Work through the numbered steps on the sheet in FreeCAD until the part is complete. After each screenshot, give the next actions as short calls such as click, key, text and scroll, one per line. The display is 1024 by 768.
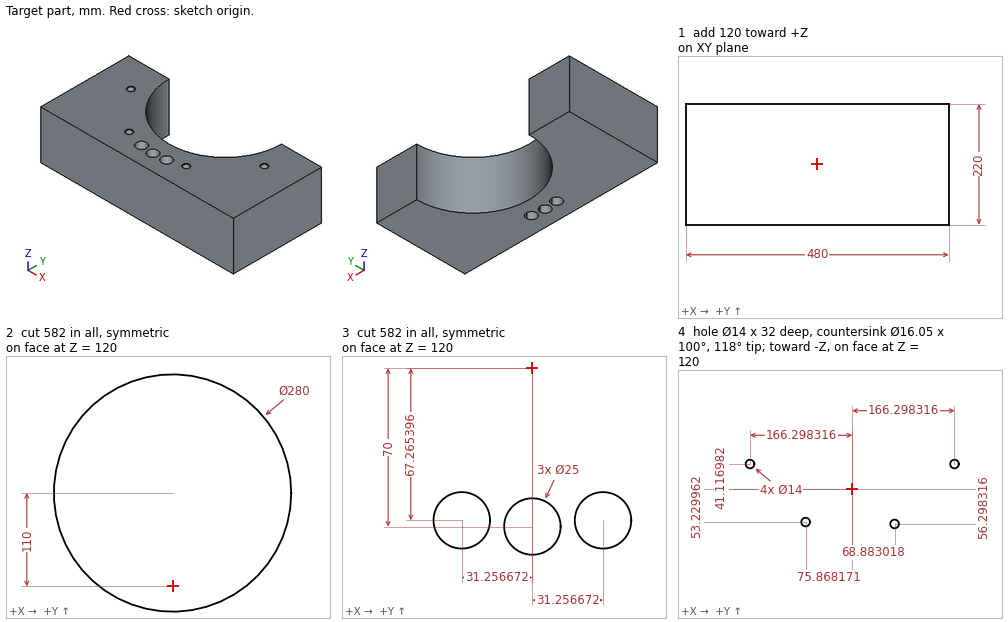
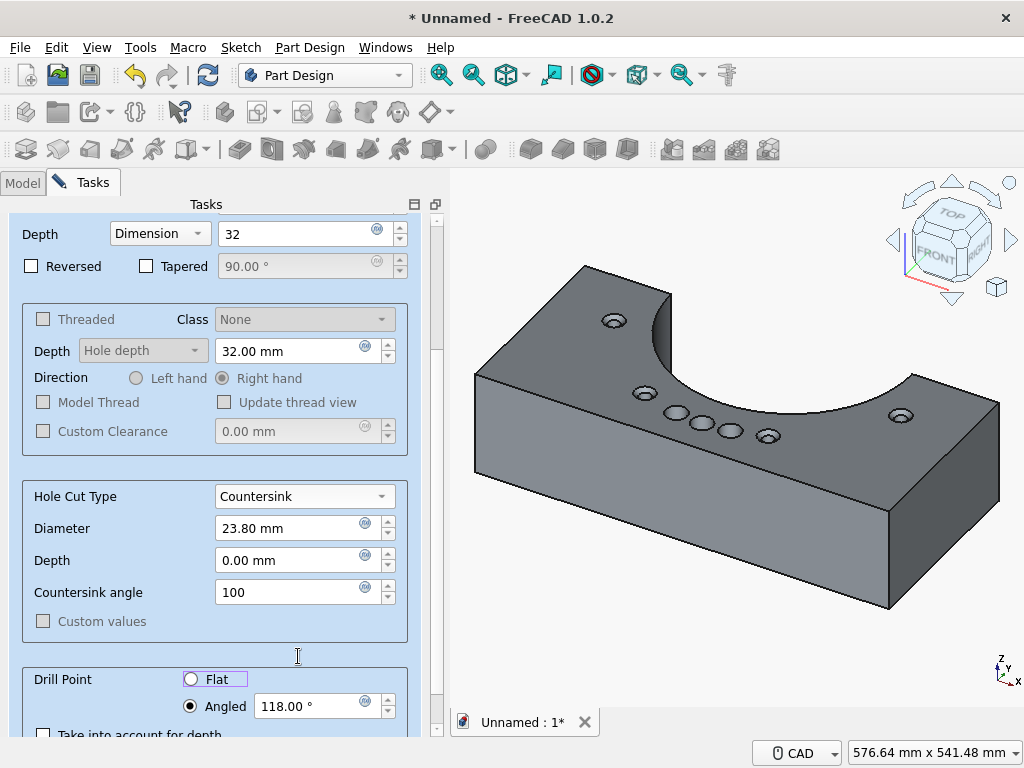
triple_click(298, 528)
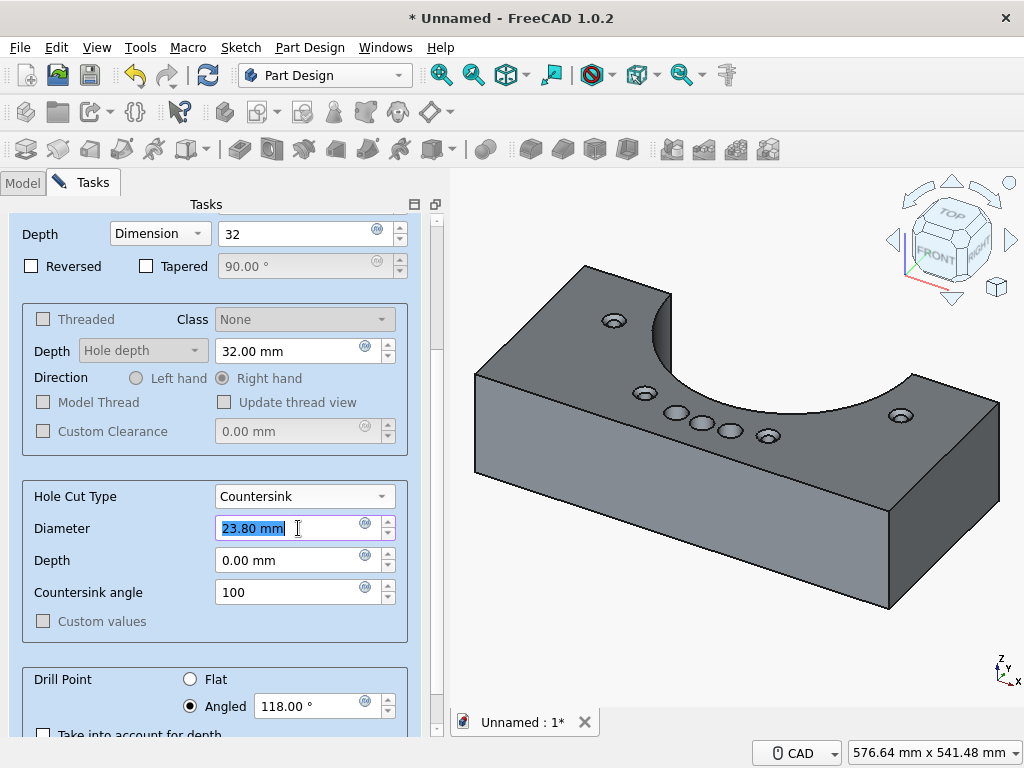
text(16.05)
key(Tab)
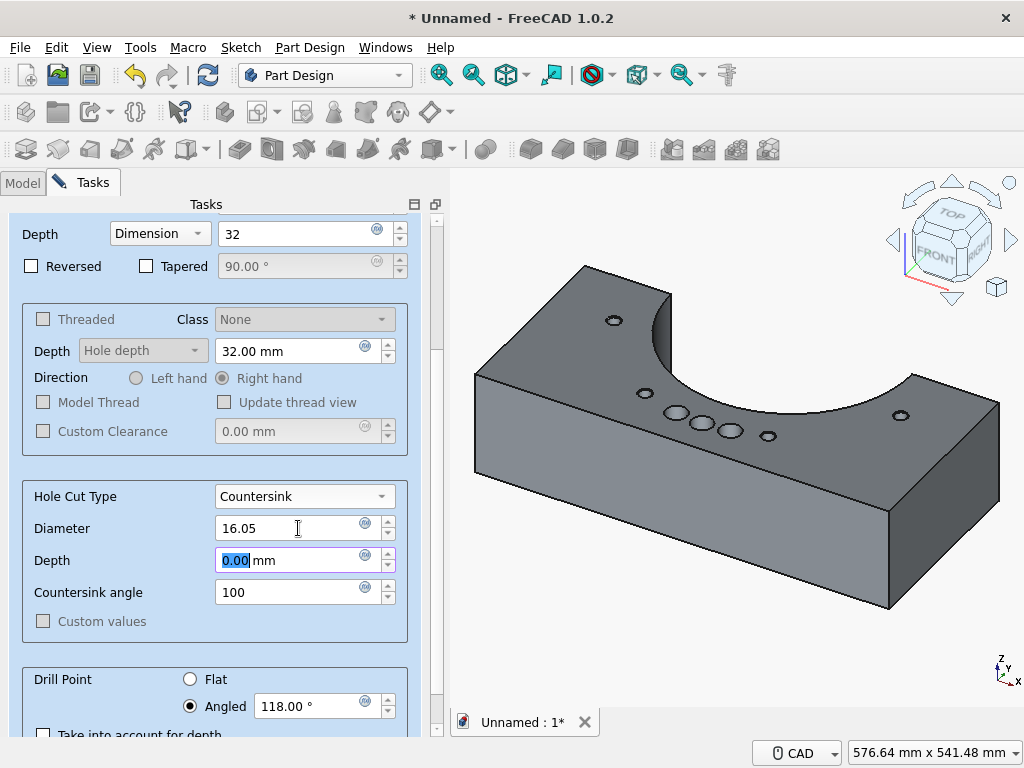
scroll(437, 475, up, 4)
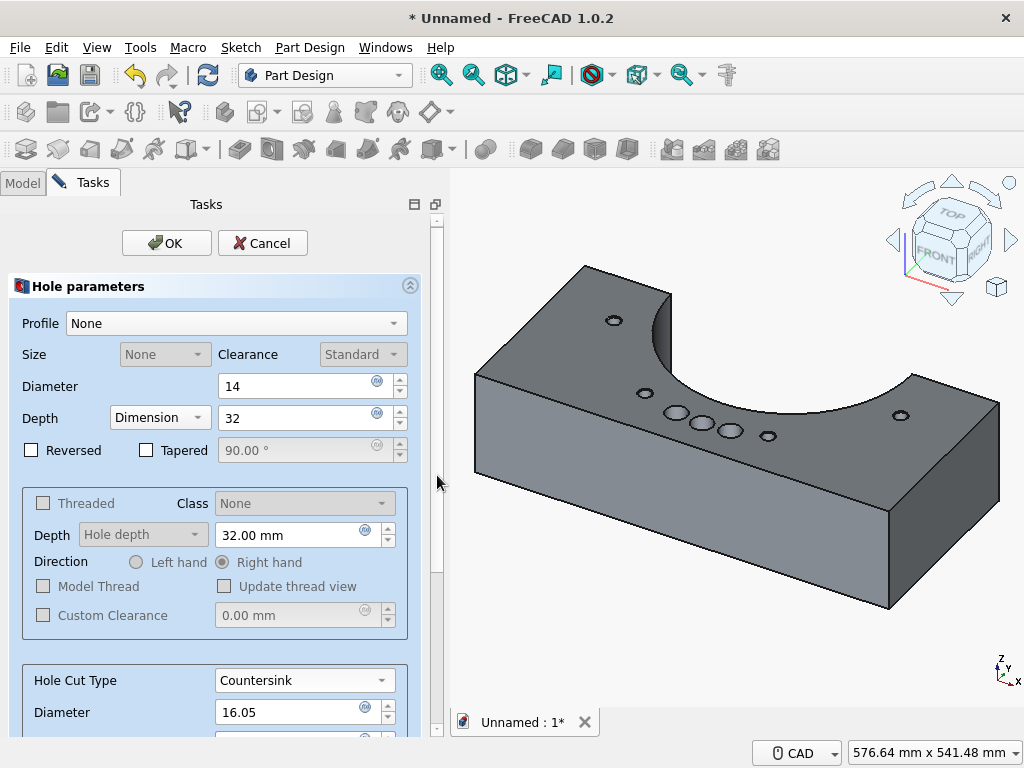
click(167, 243)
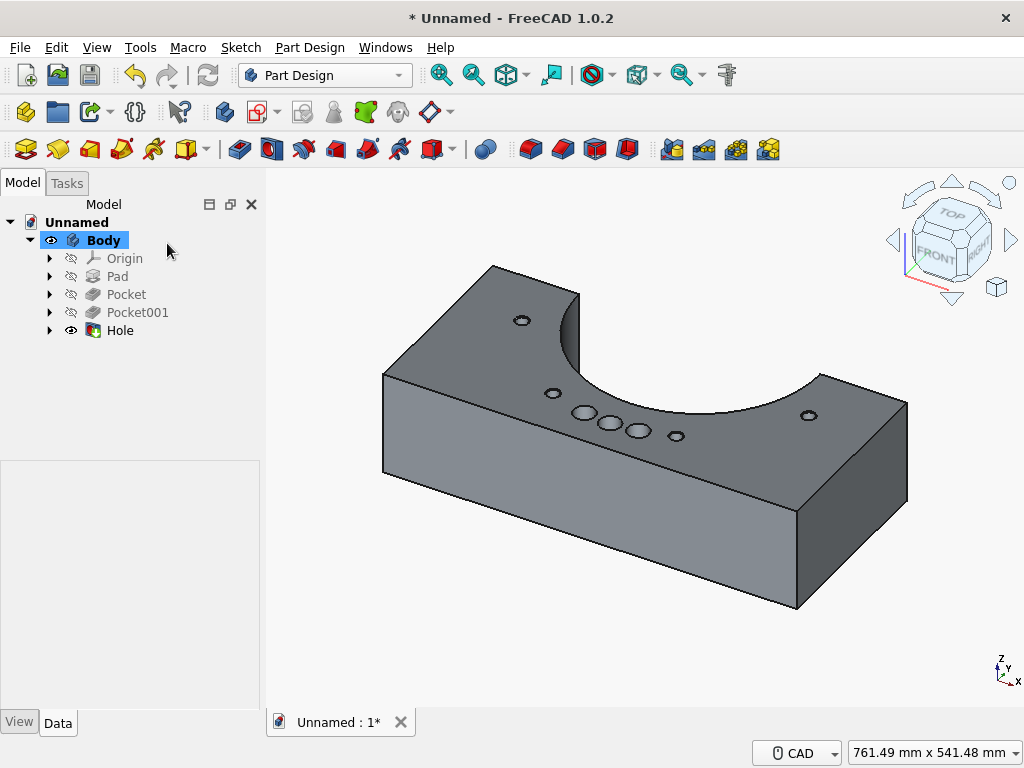
key(0)